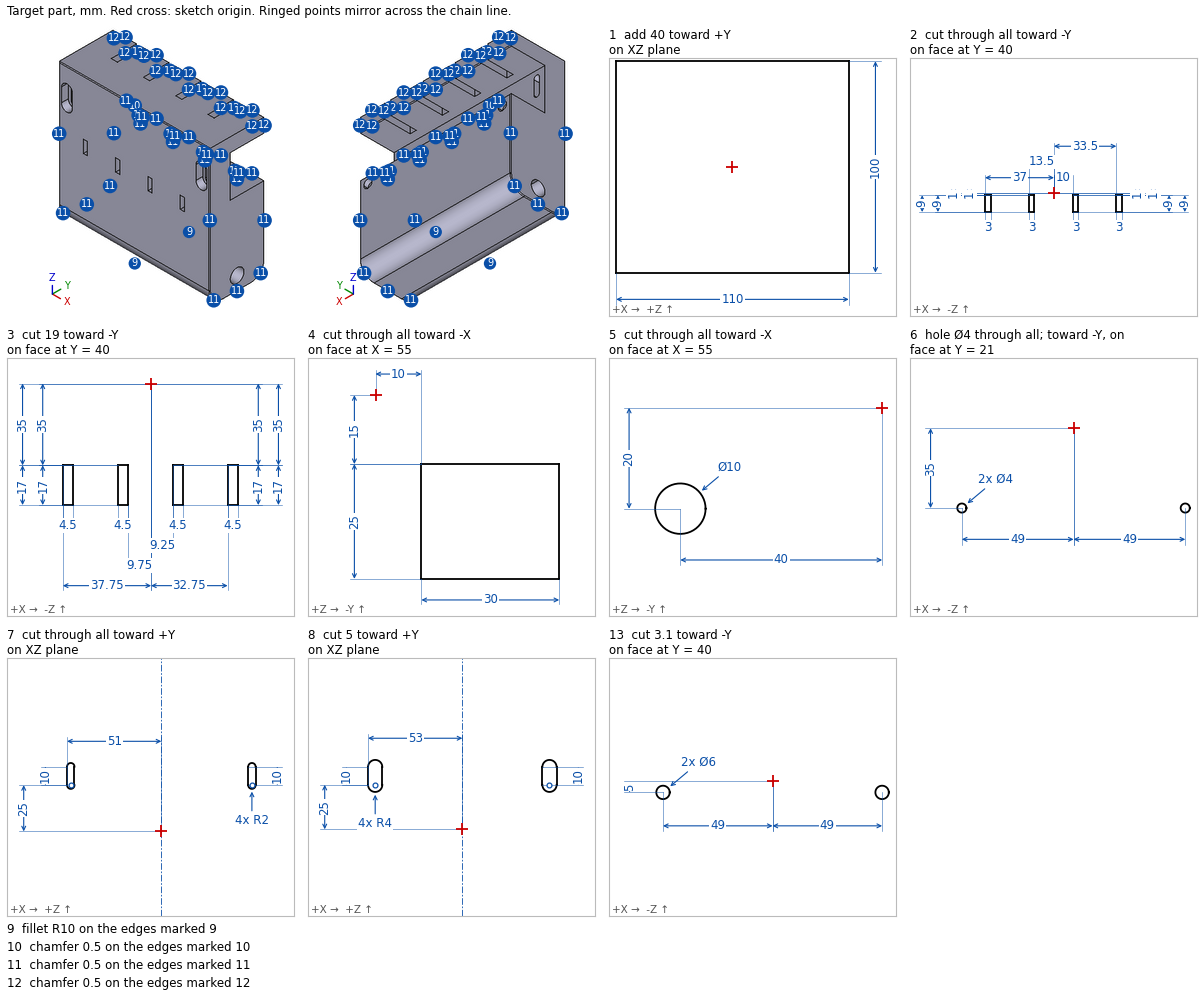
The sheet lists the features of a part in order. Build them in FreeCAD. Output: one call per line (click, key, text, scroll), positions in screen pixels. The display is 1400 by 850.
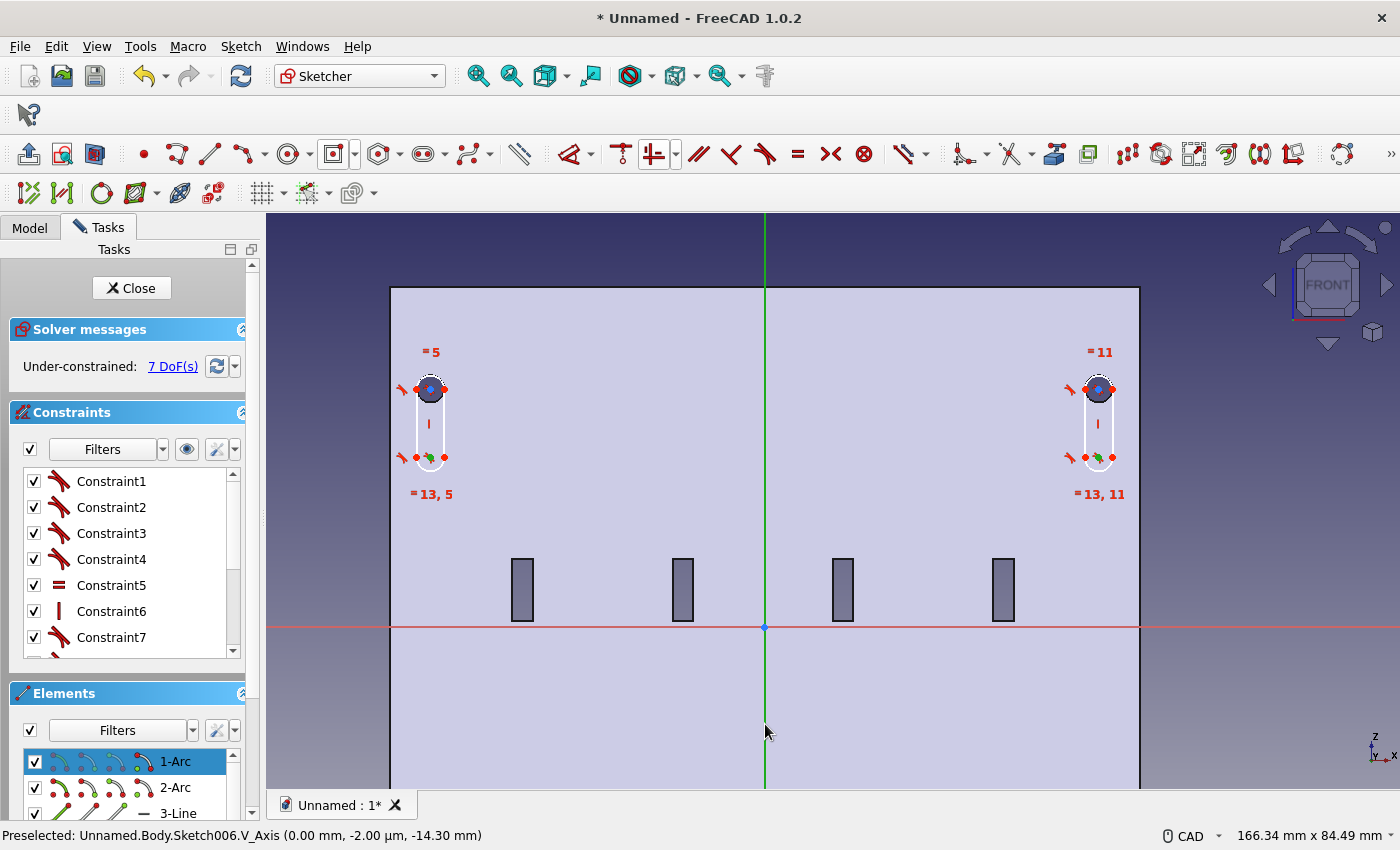
key(s)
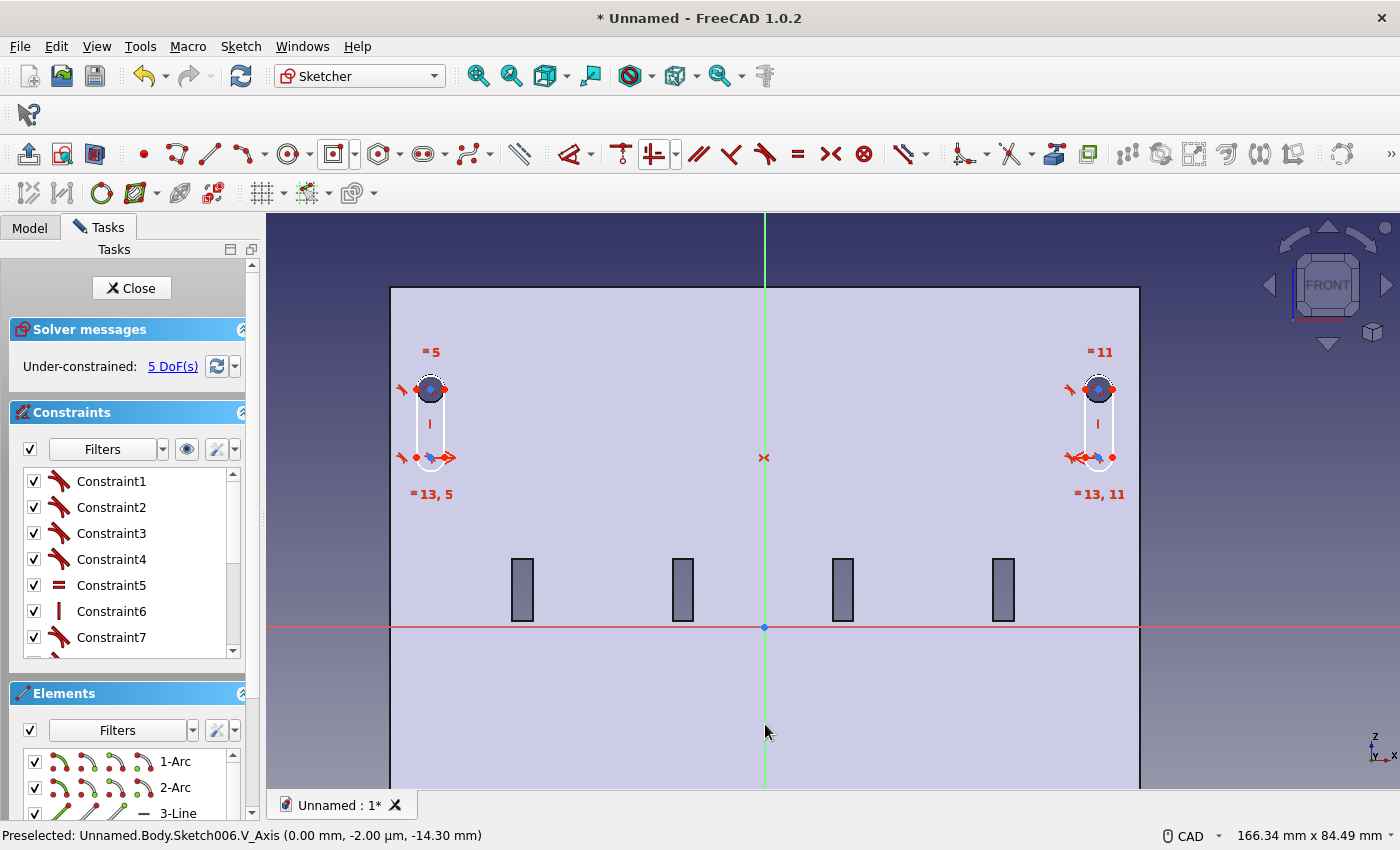
click(568, 154)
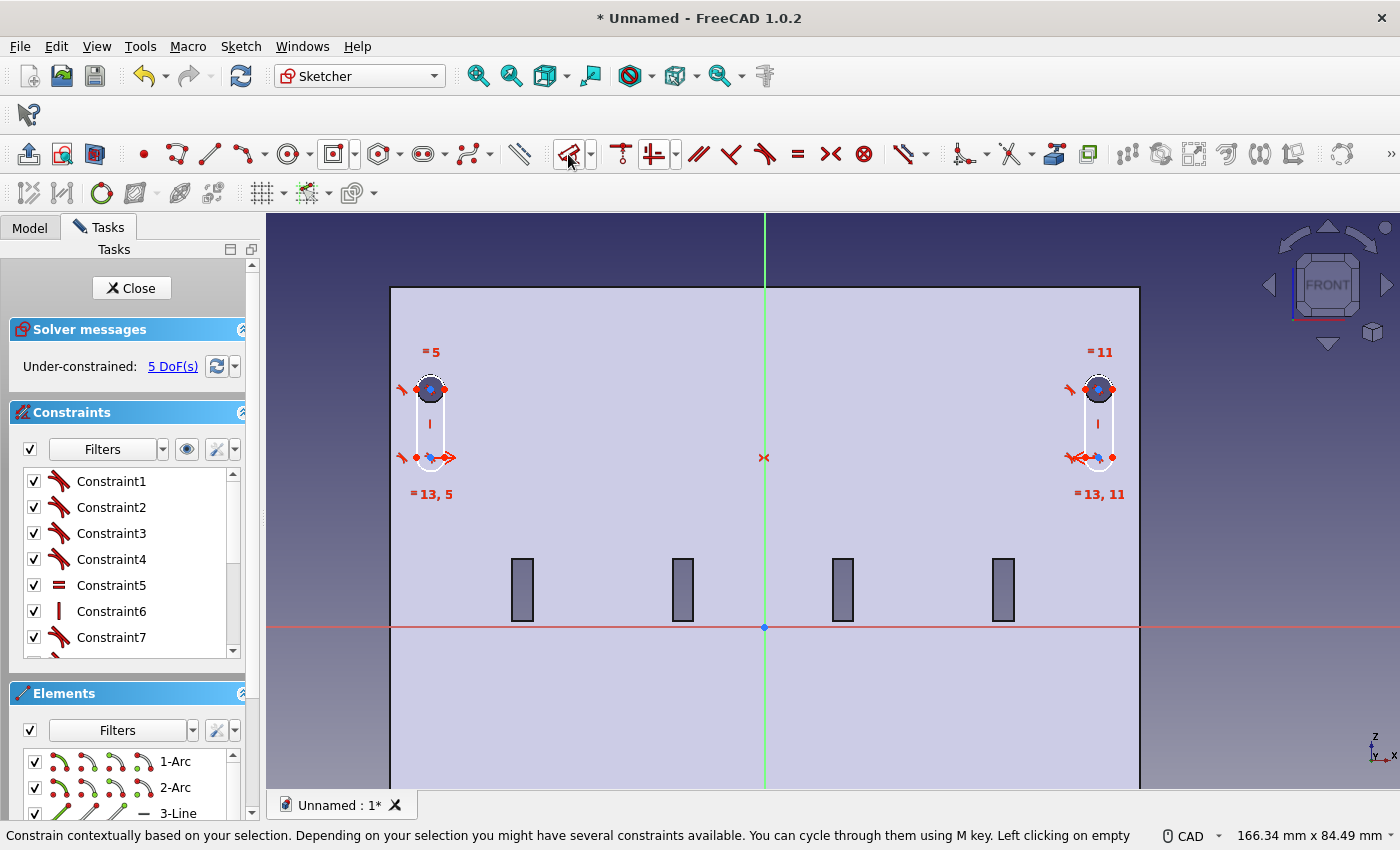
scroll(423, 469, up, 6)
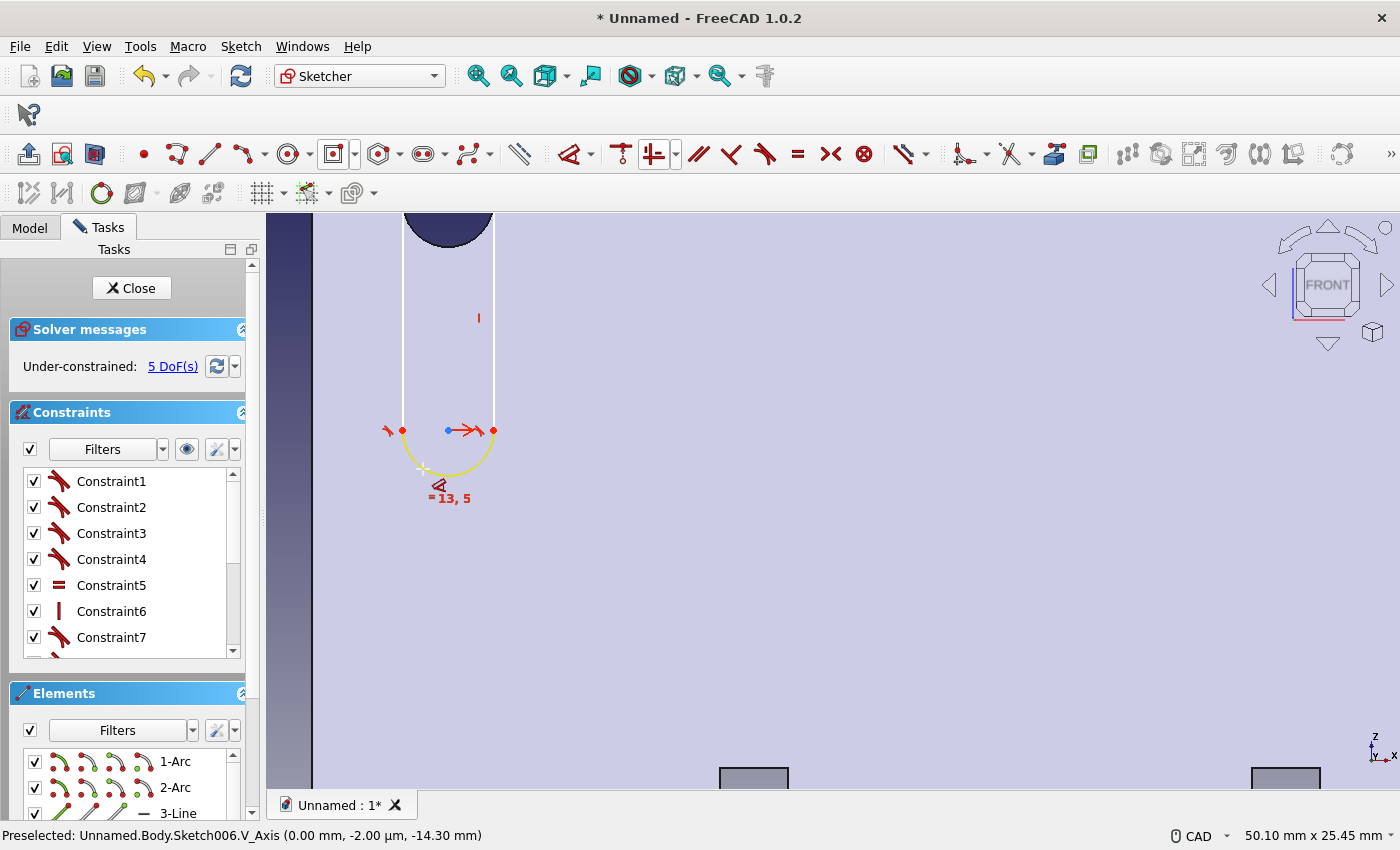
click(421, 467)
click(402, 493)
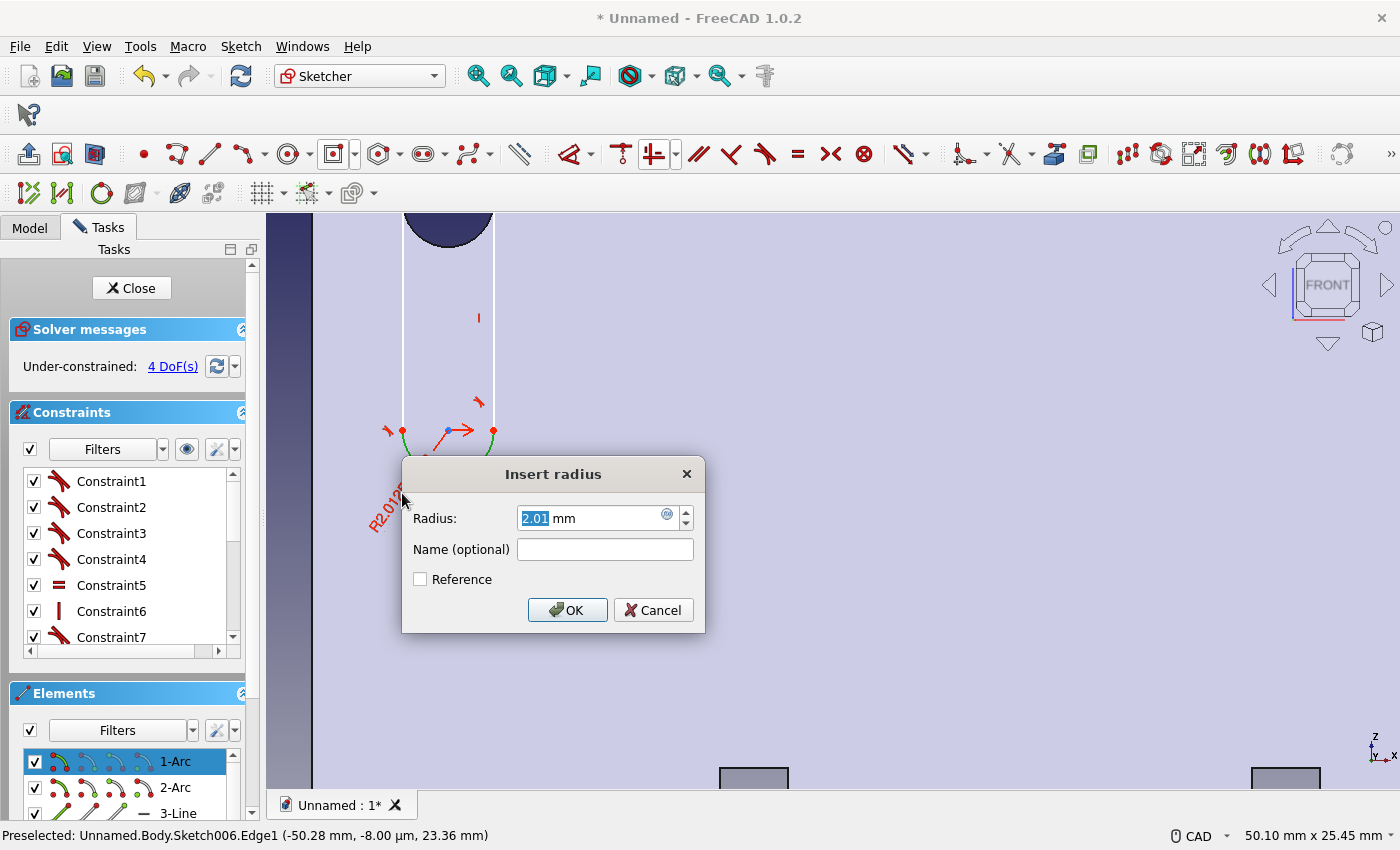
text(2)
key(Return)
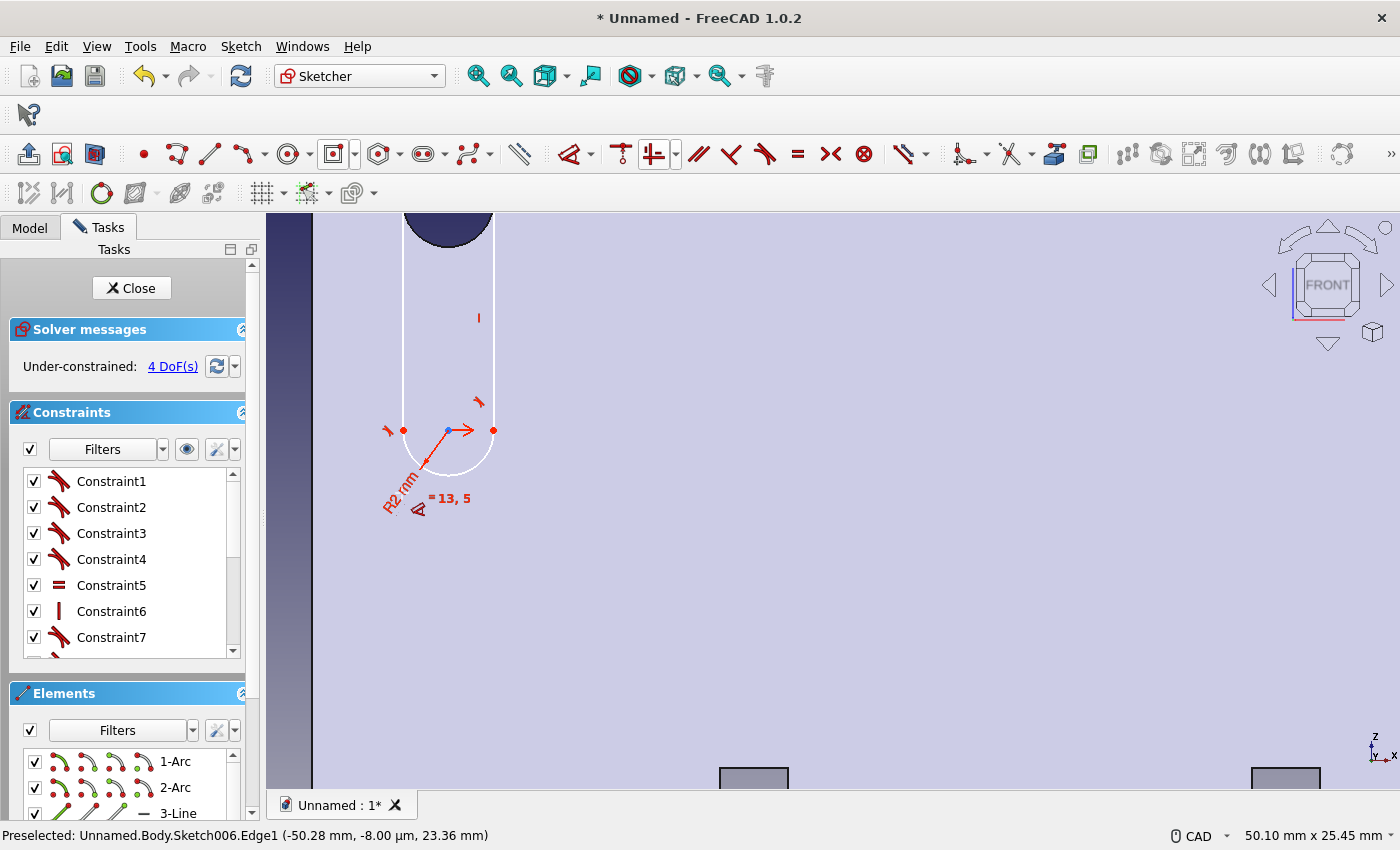
click(403, 362)
click(369, 336)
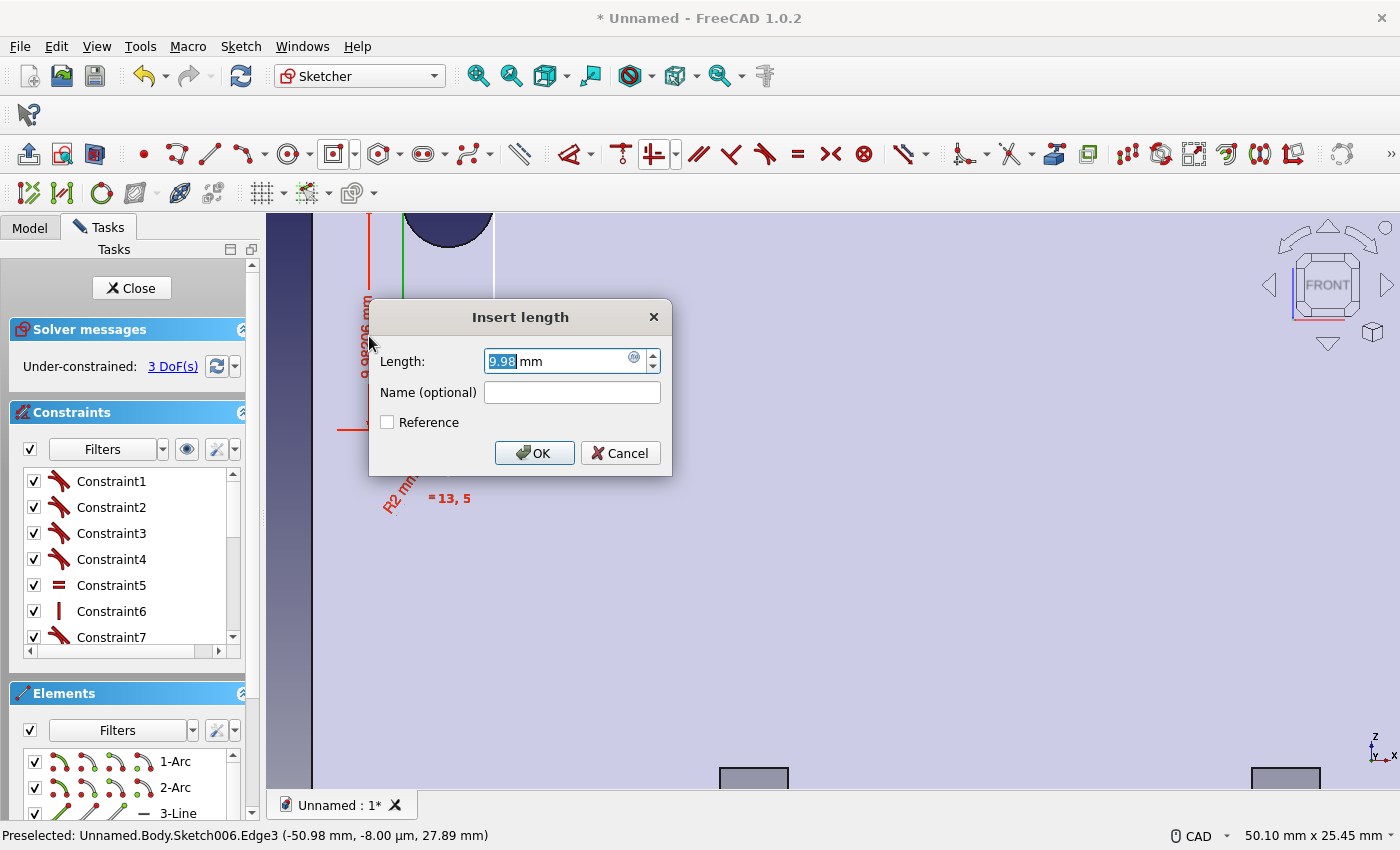
text(10)
key(Return)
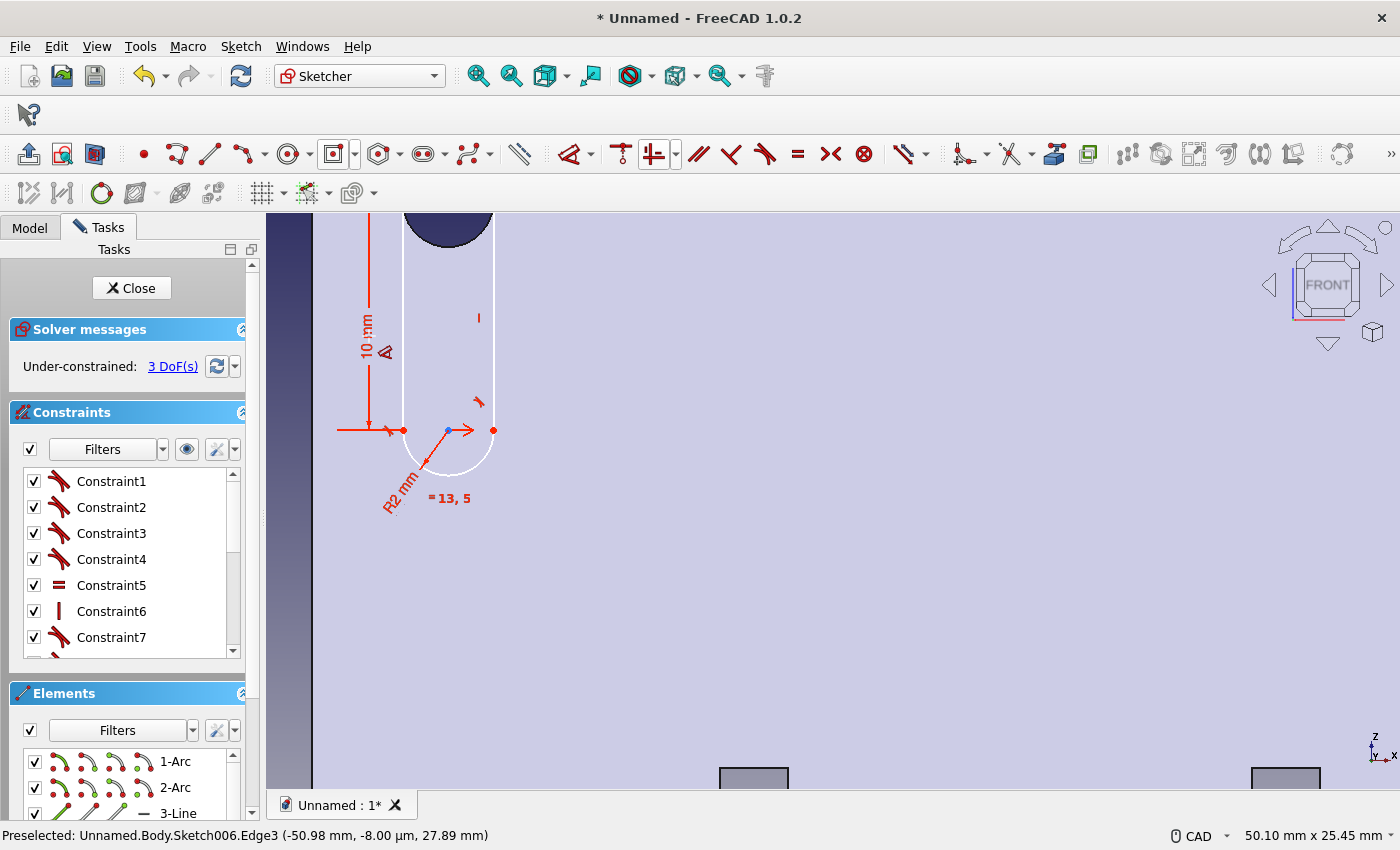
scroll(423, 469, down, 6)